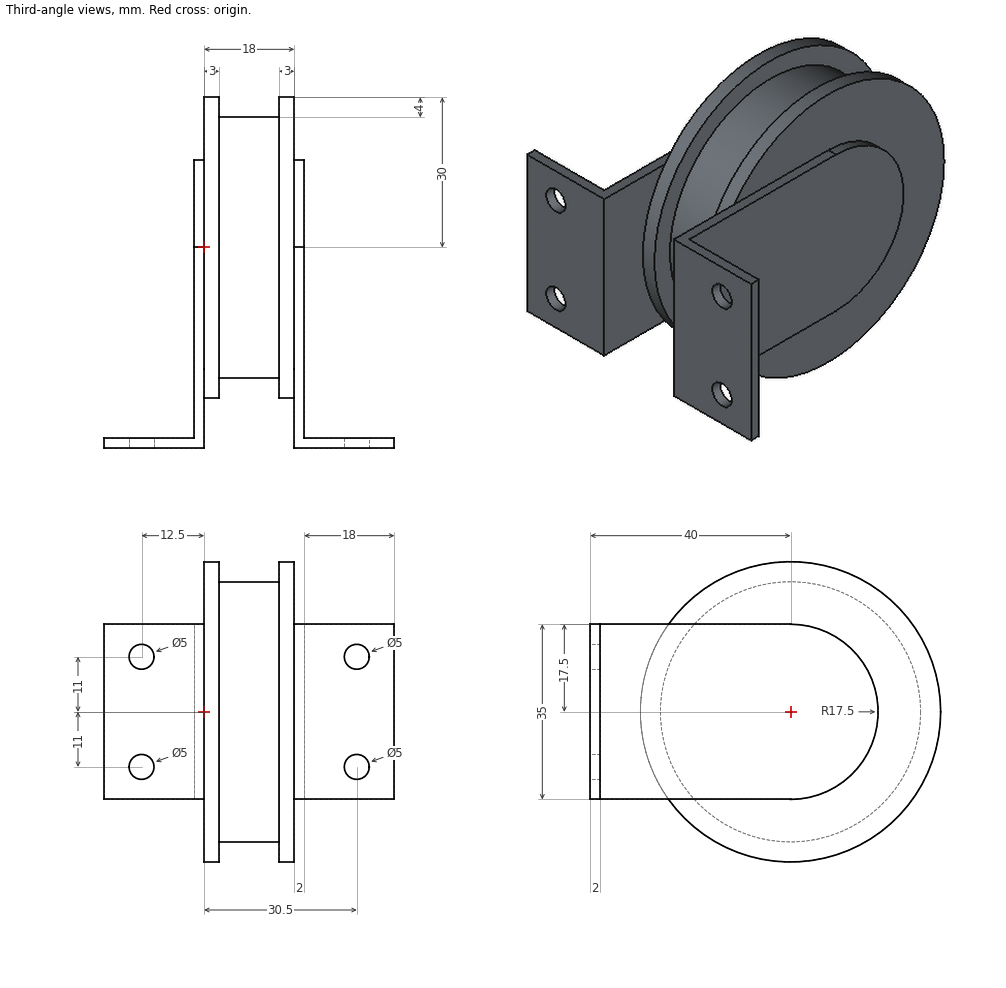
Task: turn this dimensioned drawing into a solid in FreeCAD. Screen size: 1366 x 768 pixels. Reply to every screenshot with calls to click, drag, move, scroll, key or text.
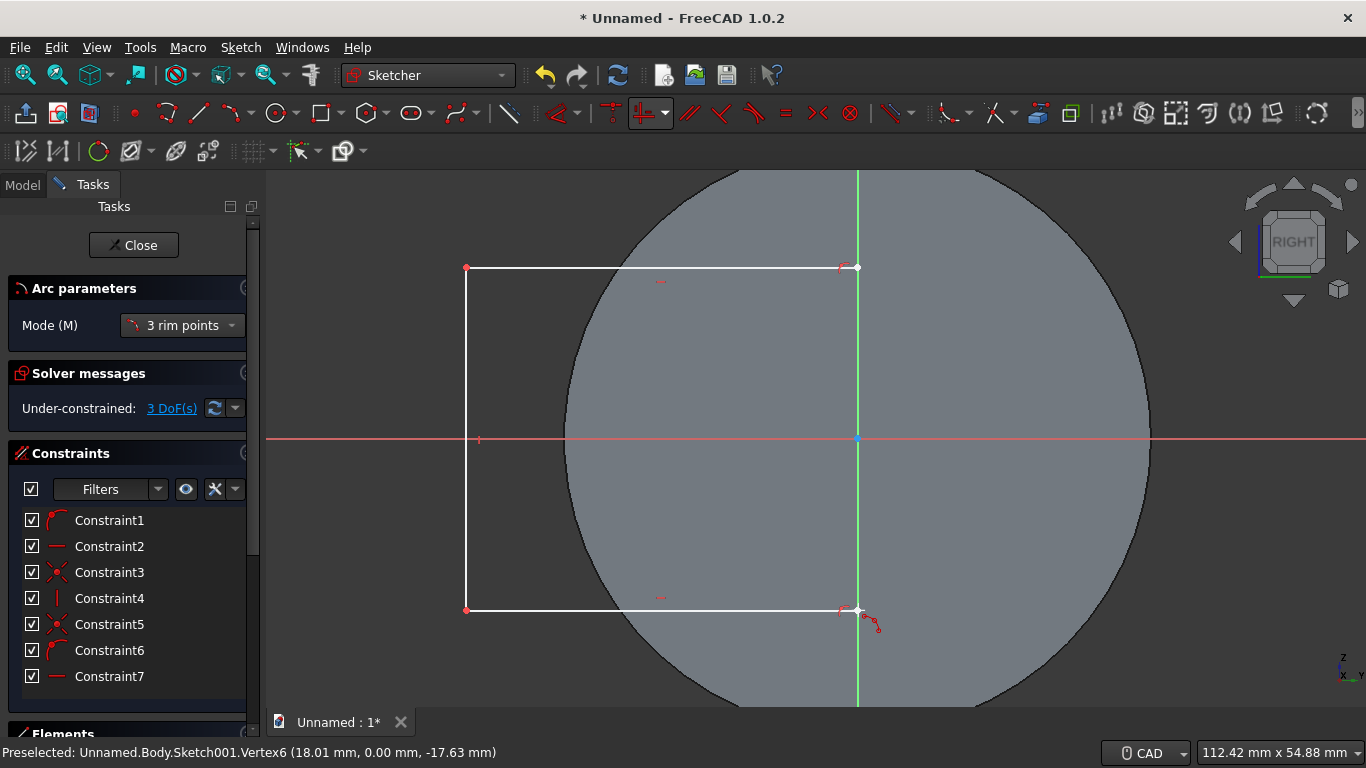
click(858, 611)
click(858, 268)
click(1020, 491)
key(Escape)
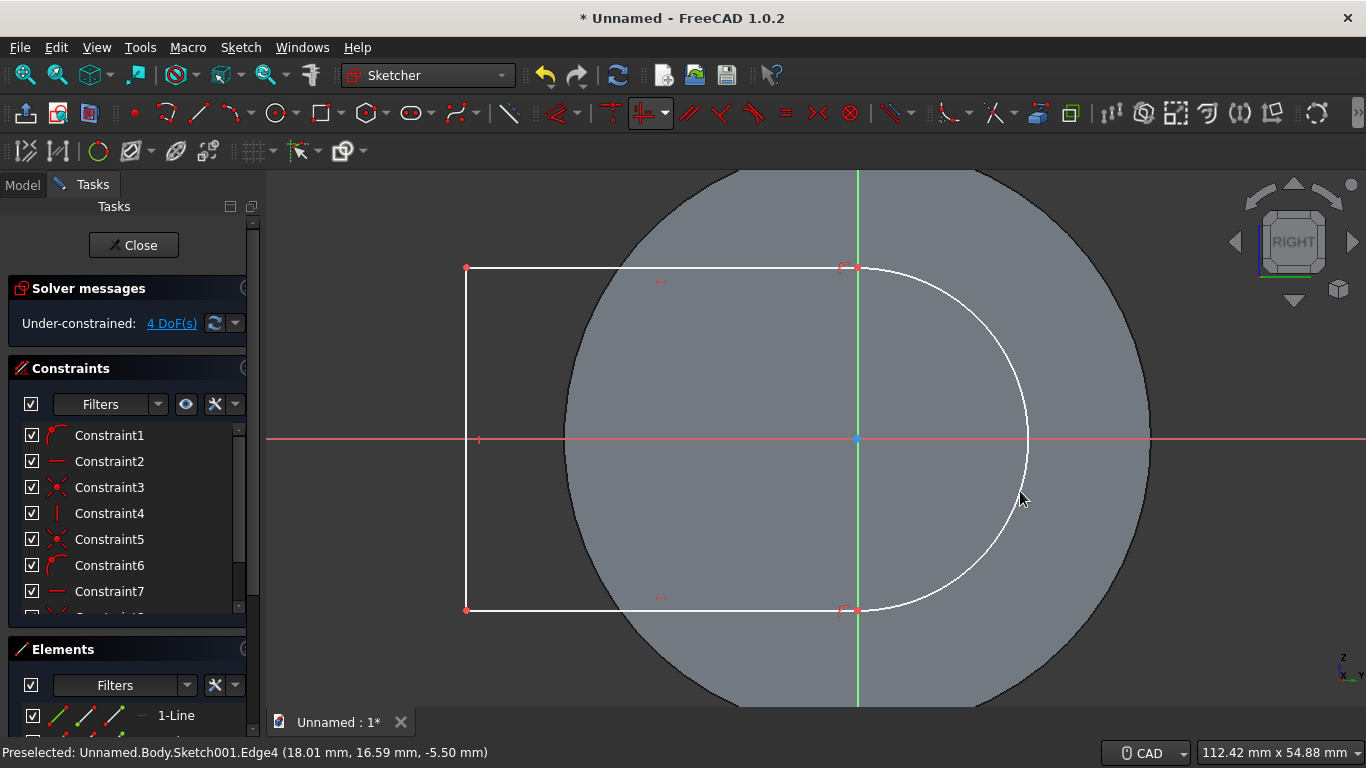
click(740, 268)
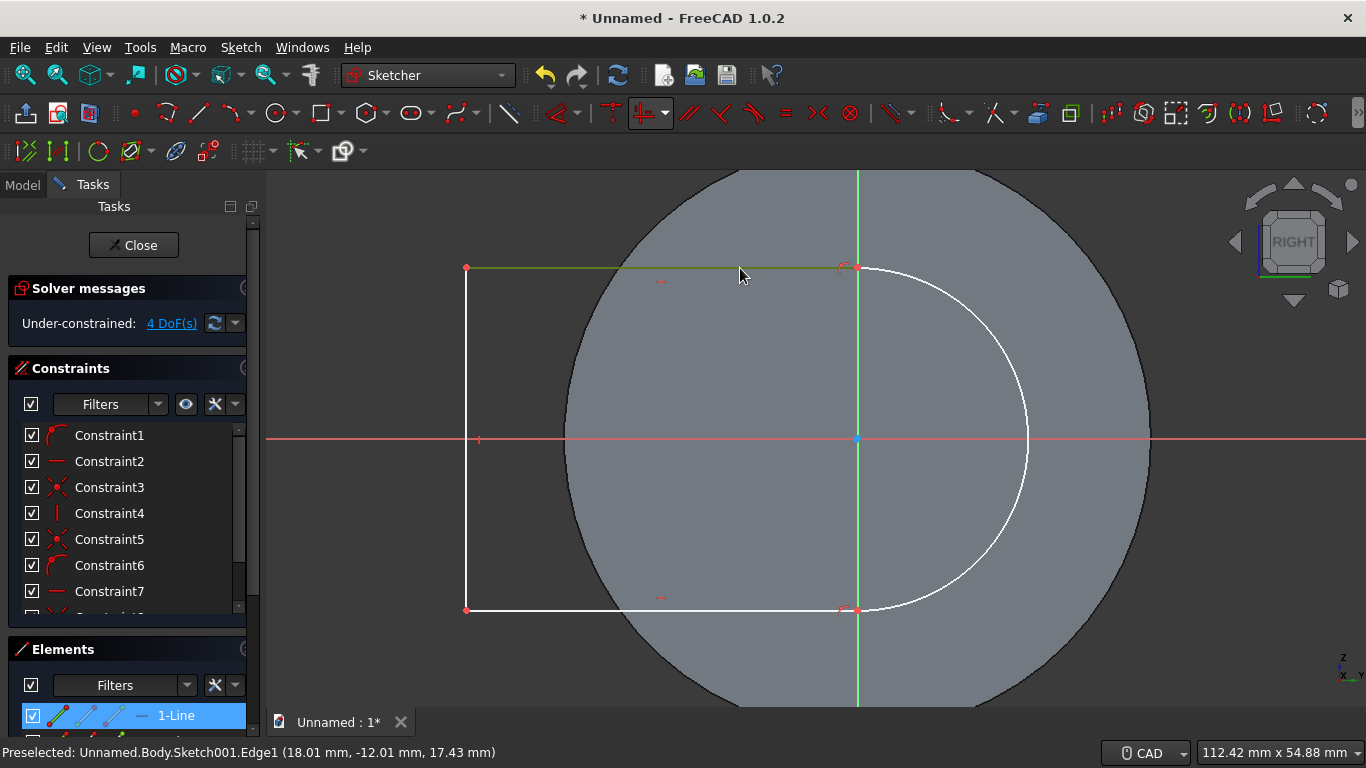
click(996, 540)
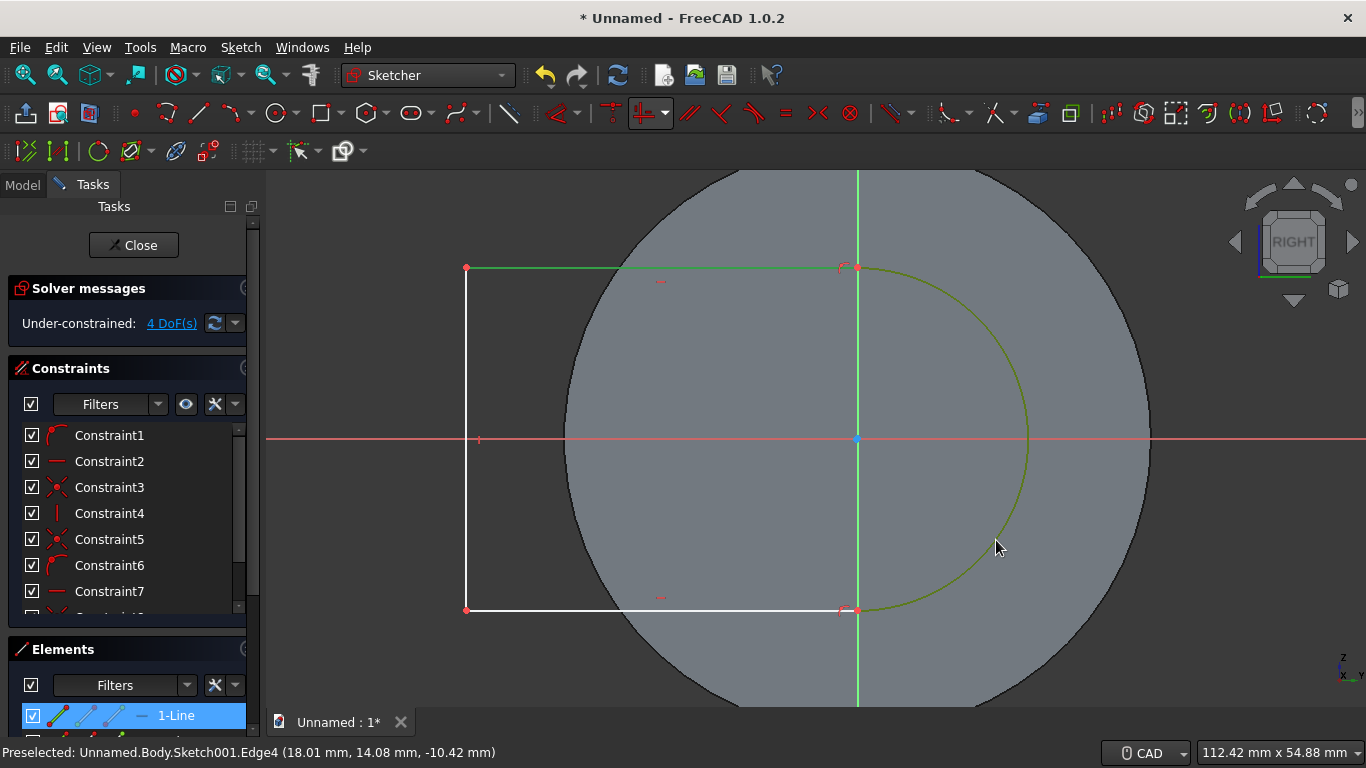
key(t)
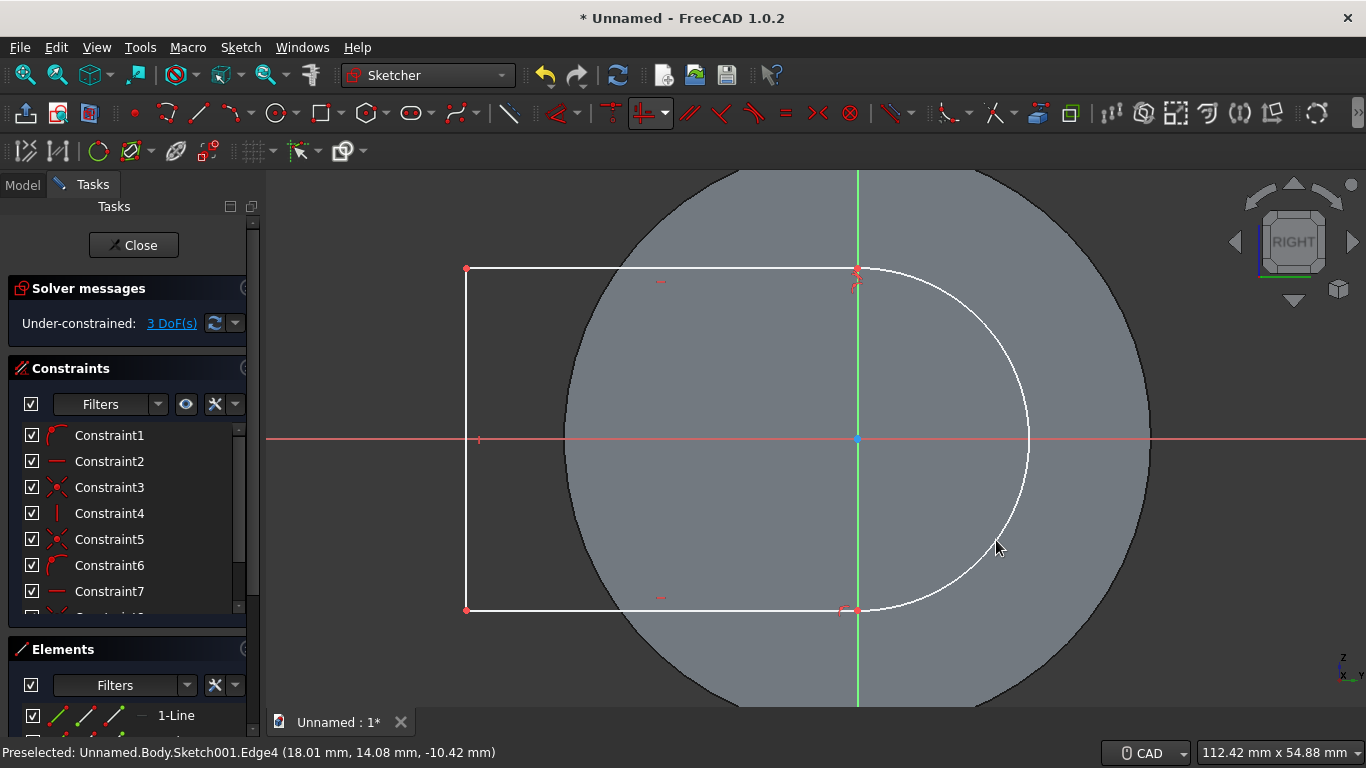
click(858, 440)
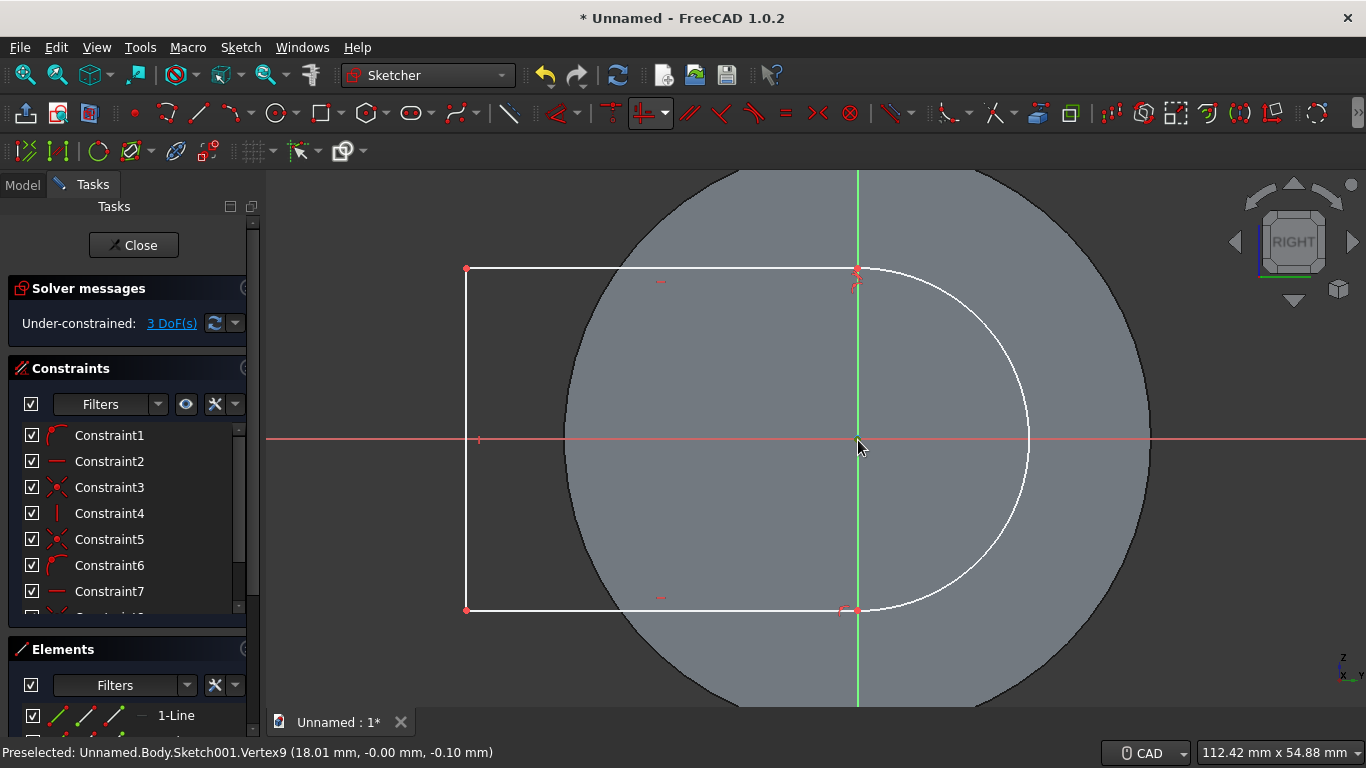
click(359, 438)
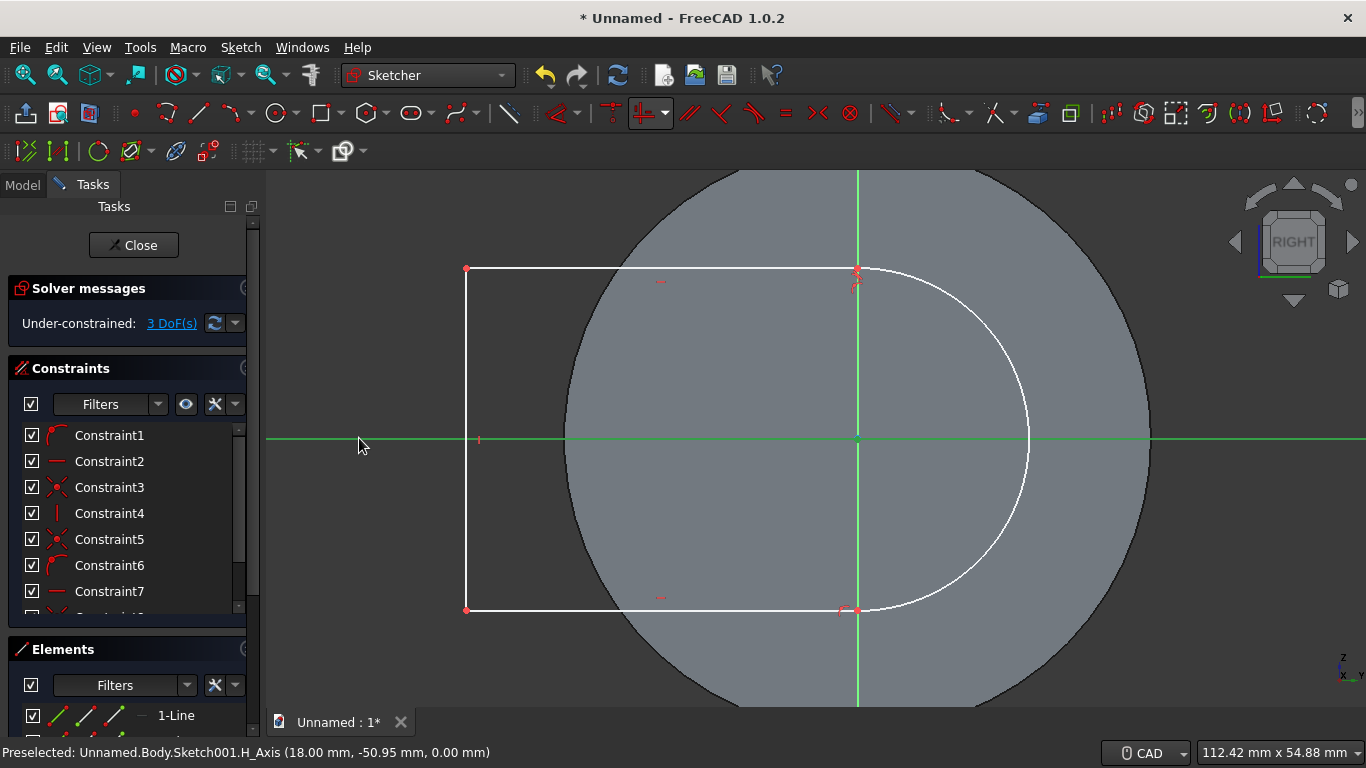
click(612, 114)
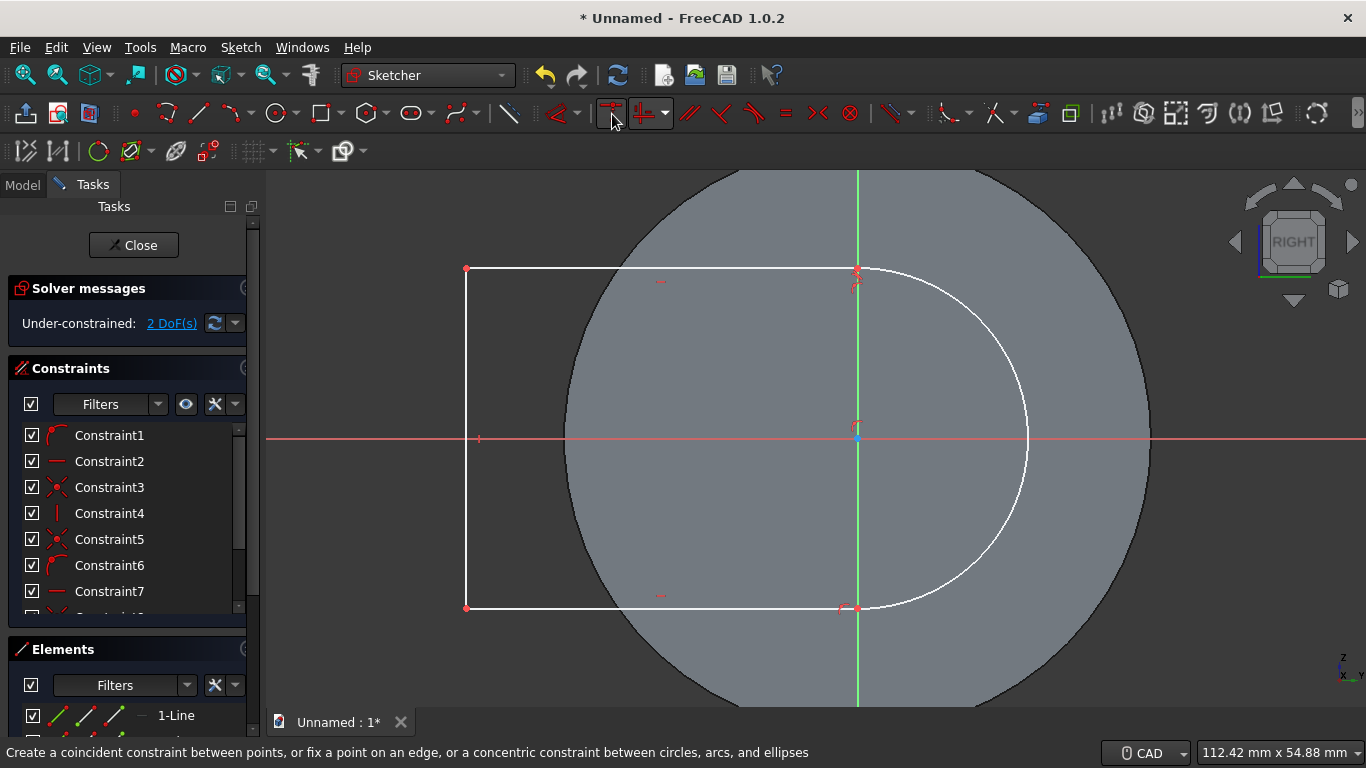
click(556, 114)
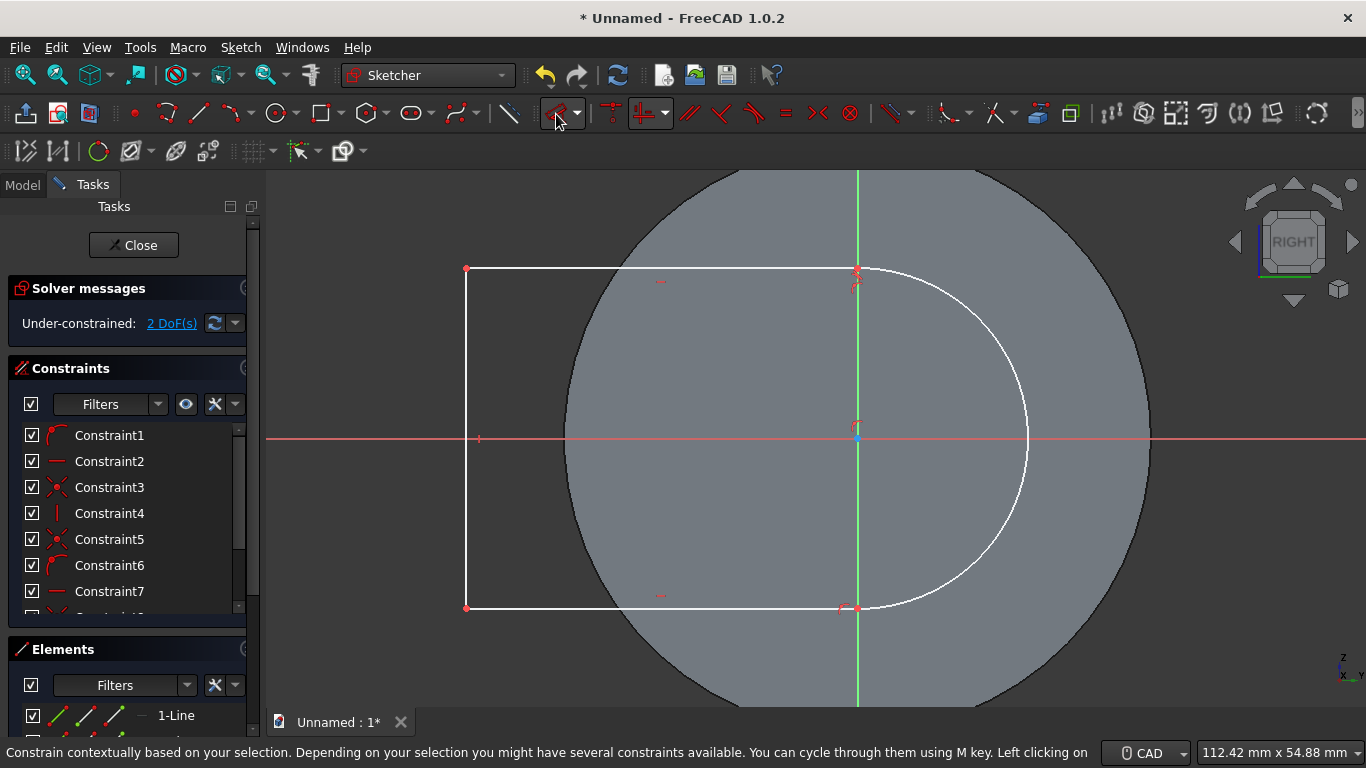
click(995, 539)
click(1021, 558)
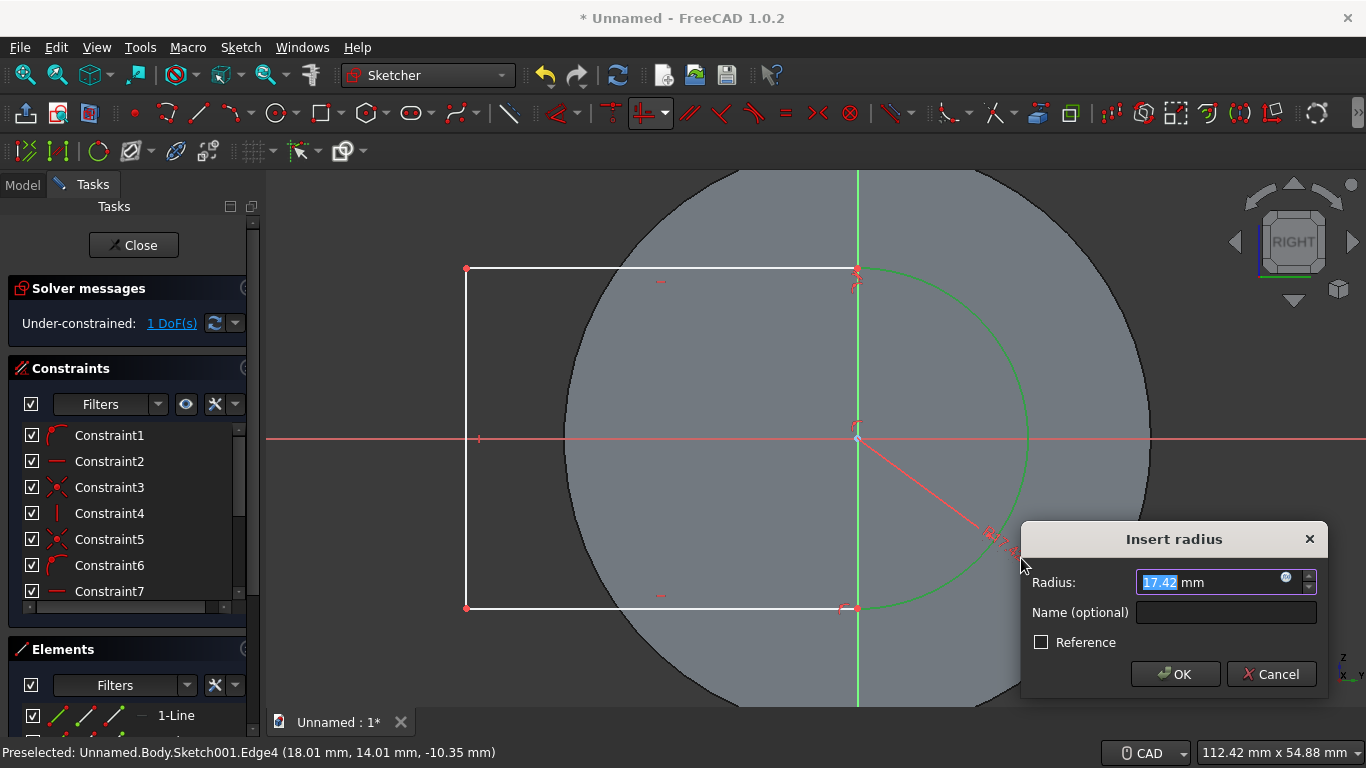
text(17.5)
key(Return)